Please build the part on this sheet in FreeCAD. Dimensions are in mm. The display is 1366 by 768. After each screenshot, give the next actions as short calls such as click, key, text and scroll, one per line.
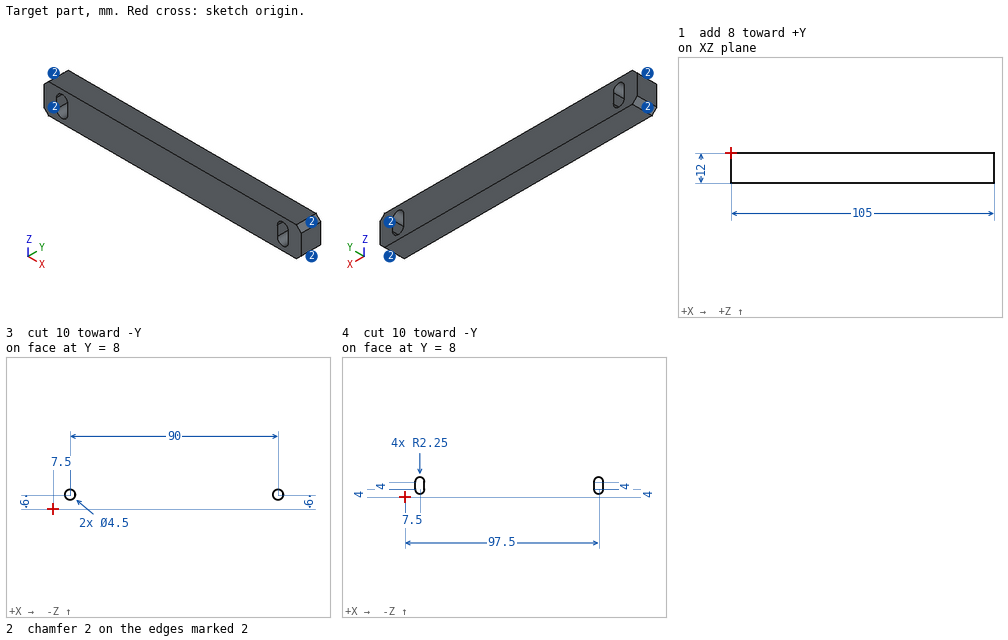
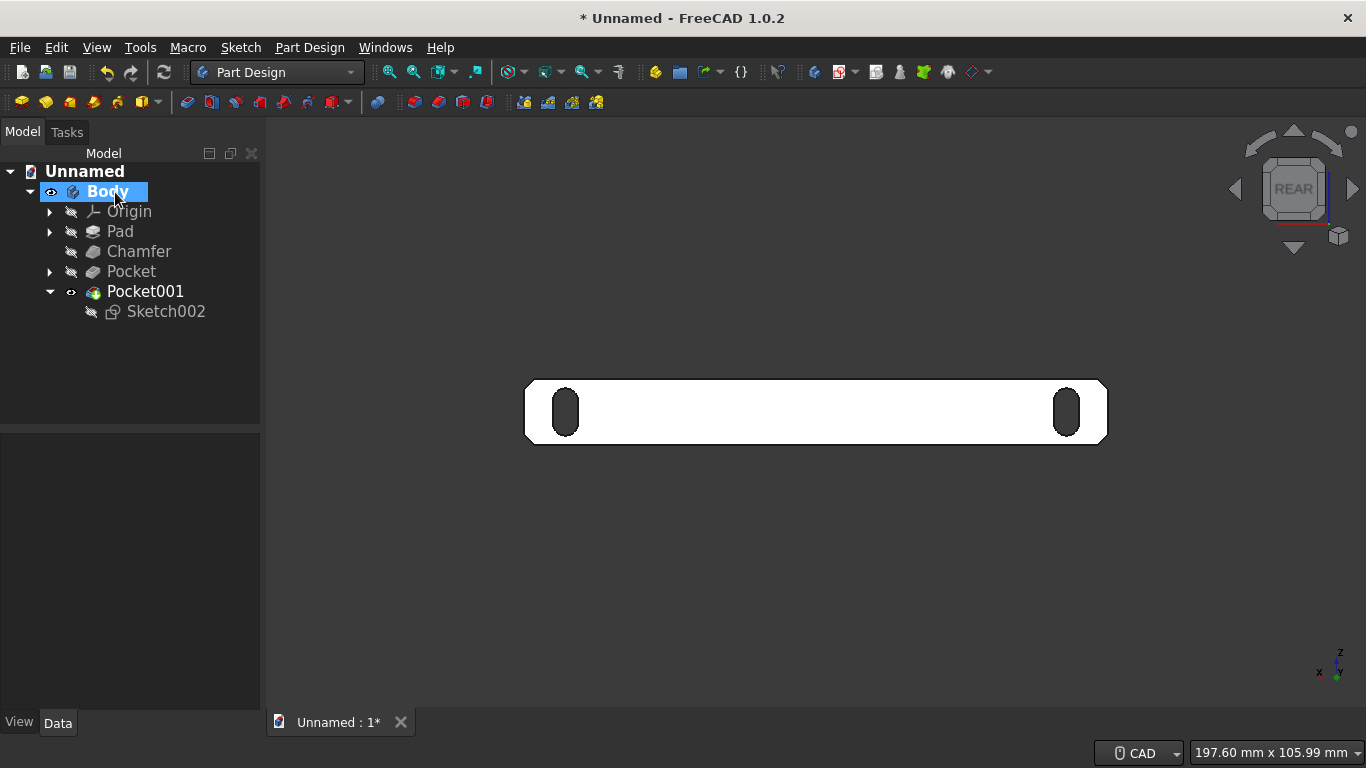
key(0)